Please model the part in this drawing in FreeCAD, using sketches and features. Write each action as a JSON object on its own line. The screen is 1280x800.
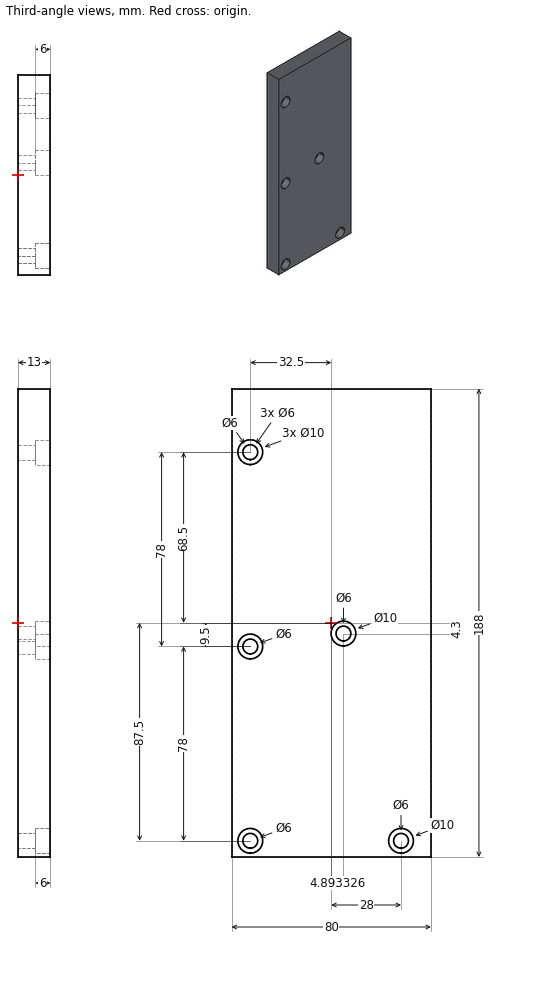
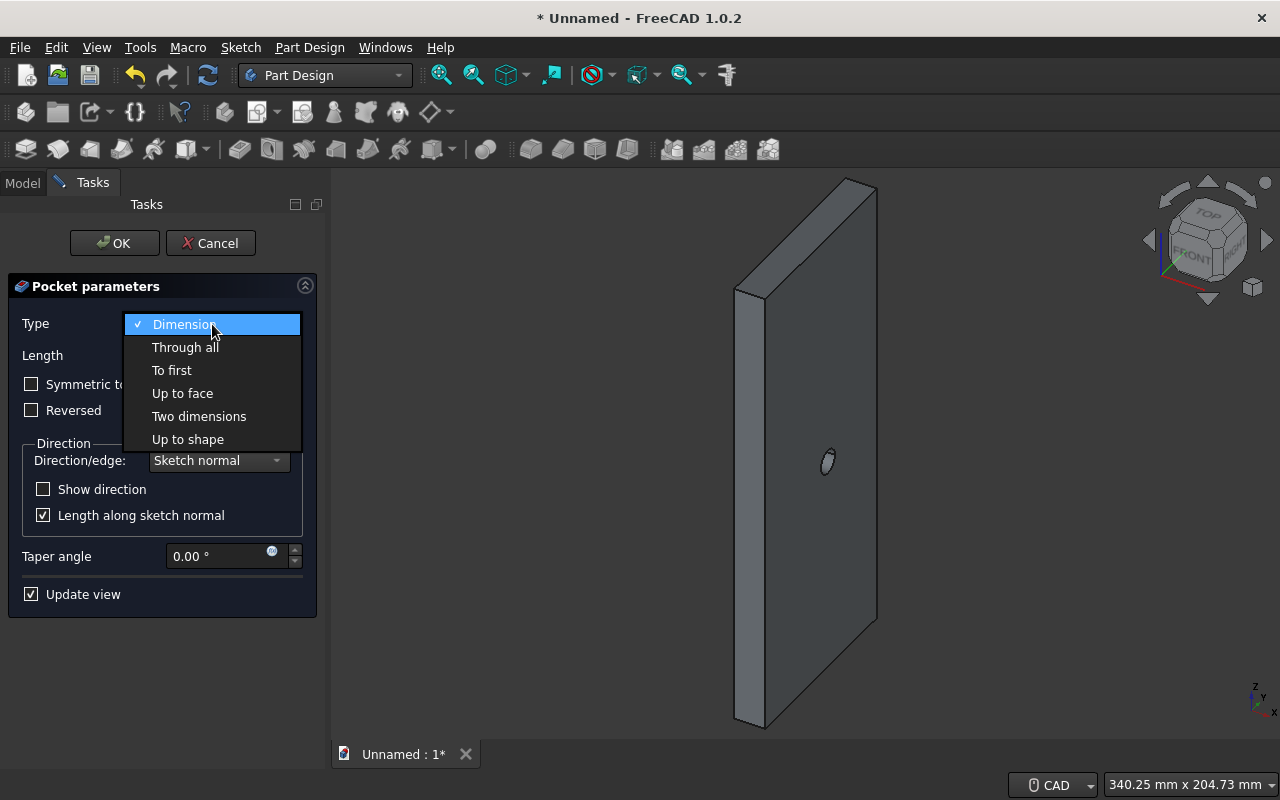
{"action": "left_click", "coordinate": [212, 370]}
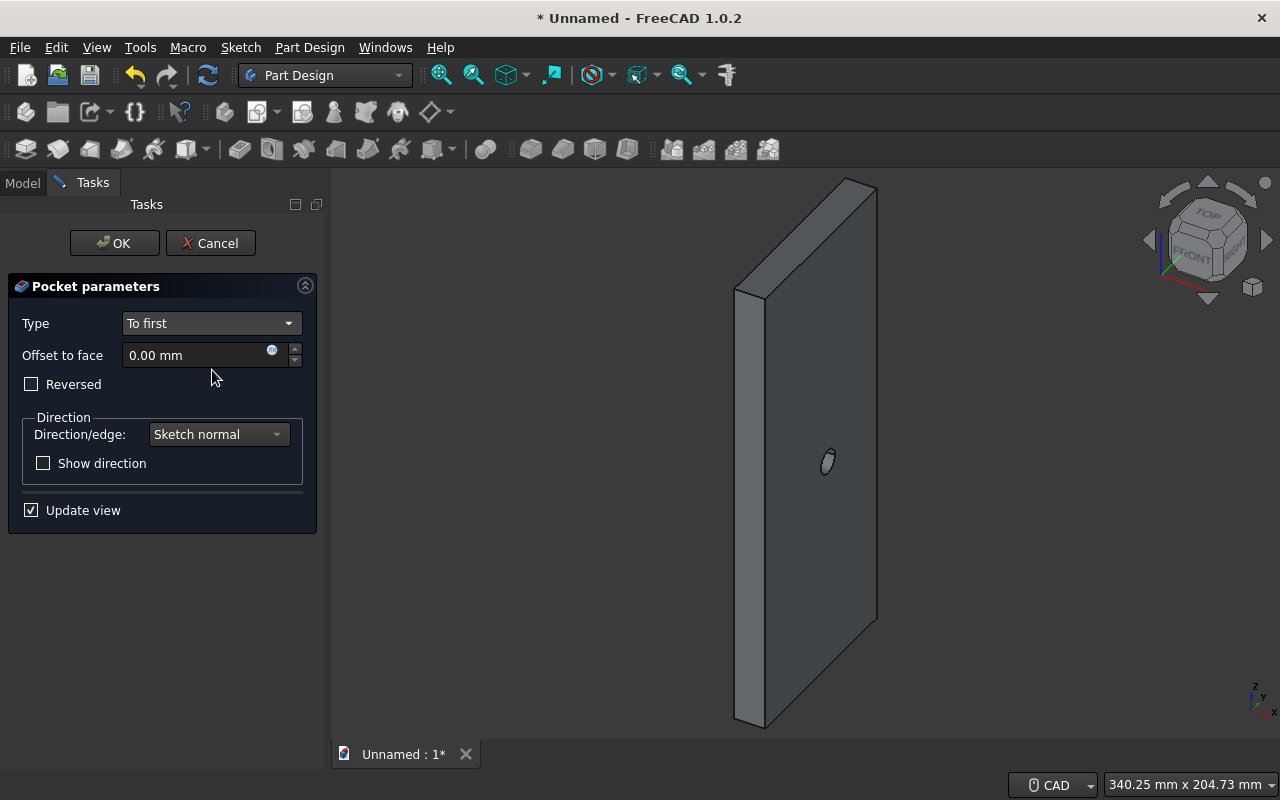
{"action": "left_click", "coordinate": [115, 243]}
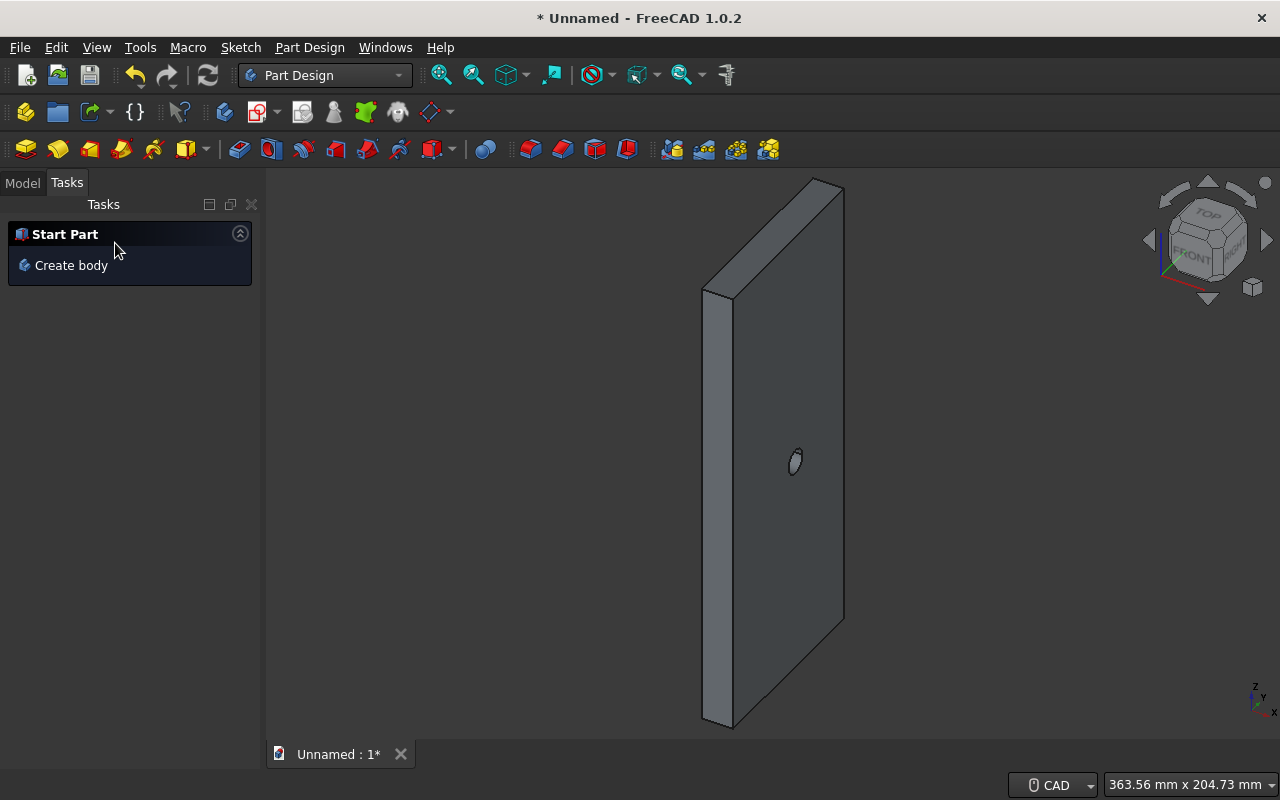
{"action": "left_click", "coordinate": [789, 580]}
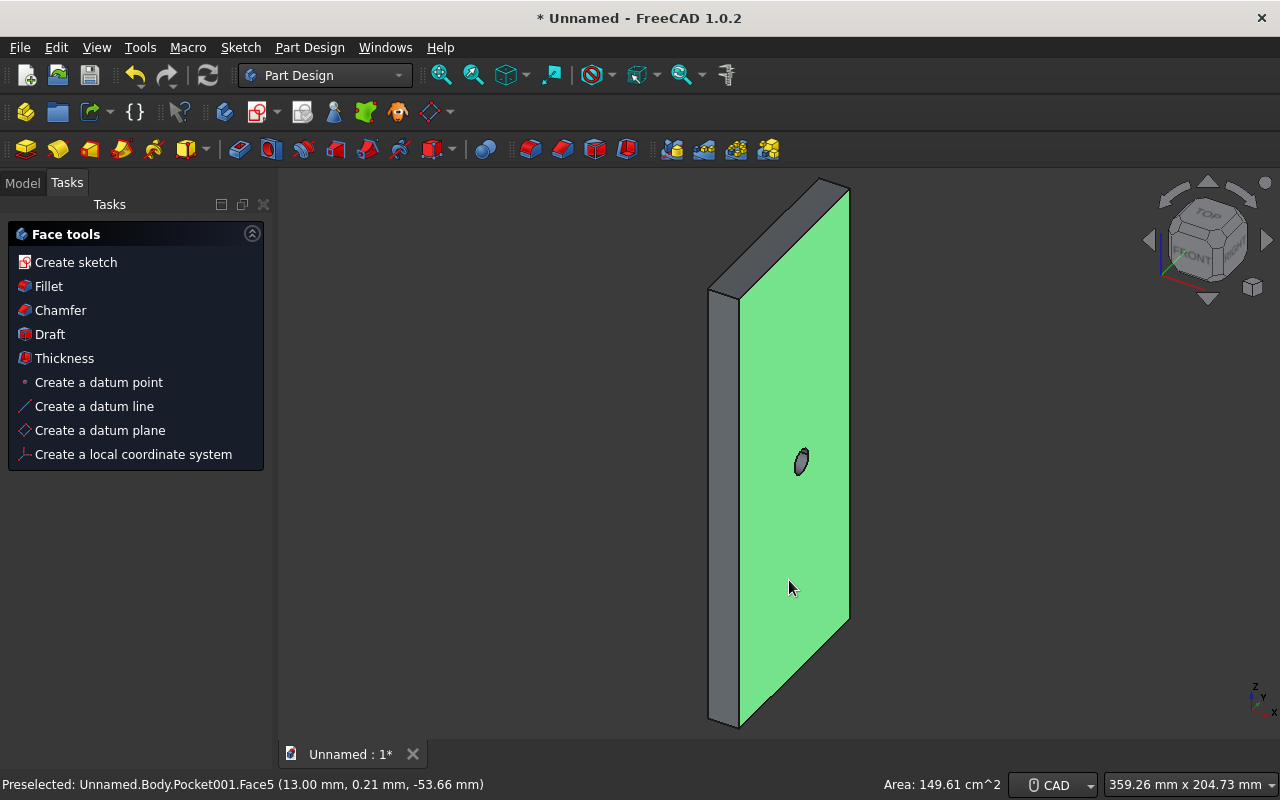
{"action": "left_click", "coordinate": [258, 112]}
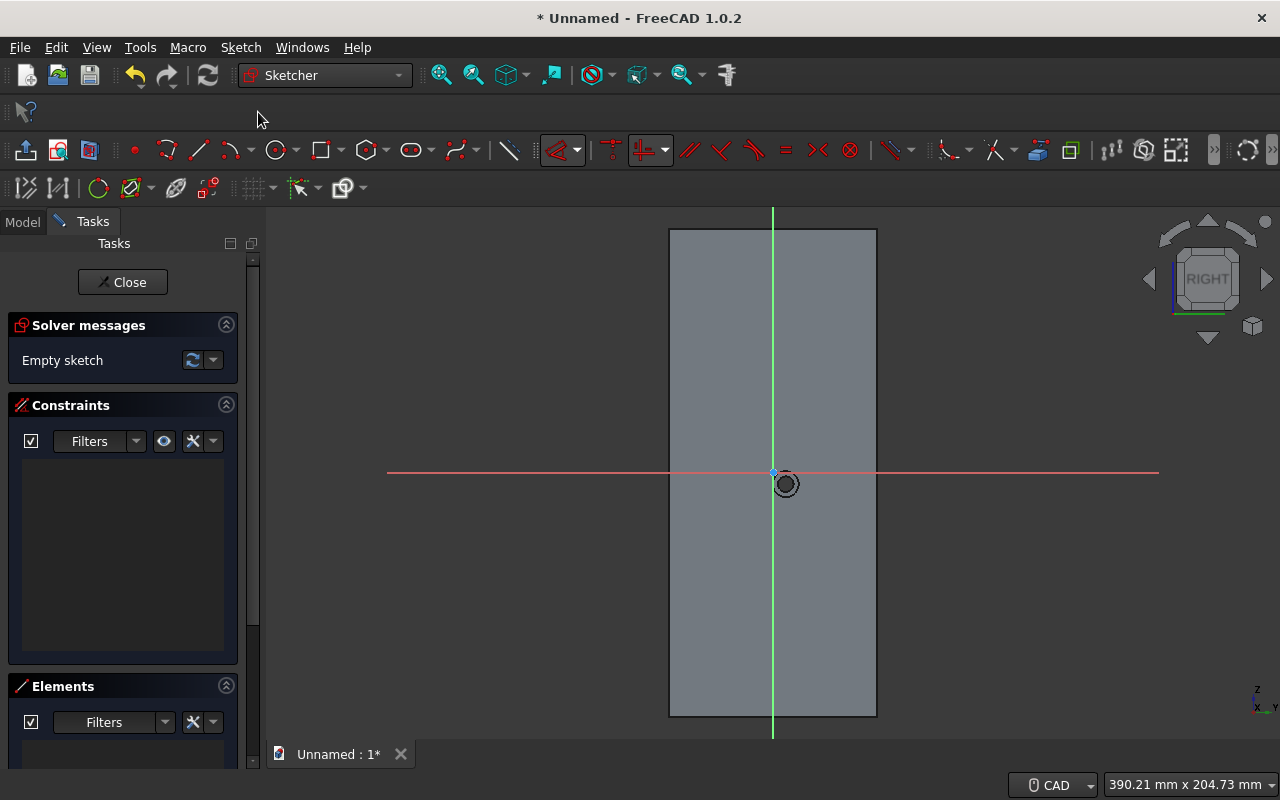
{"action": "scroll", "coordinate": [615, 361], "scroll_direction": "down", "scroll_amount": 1}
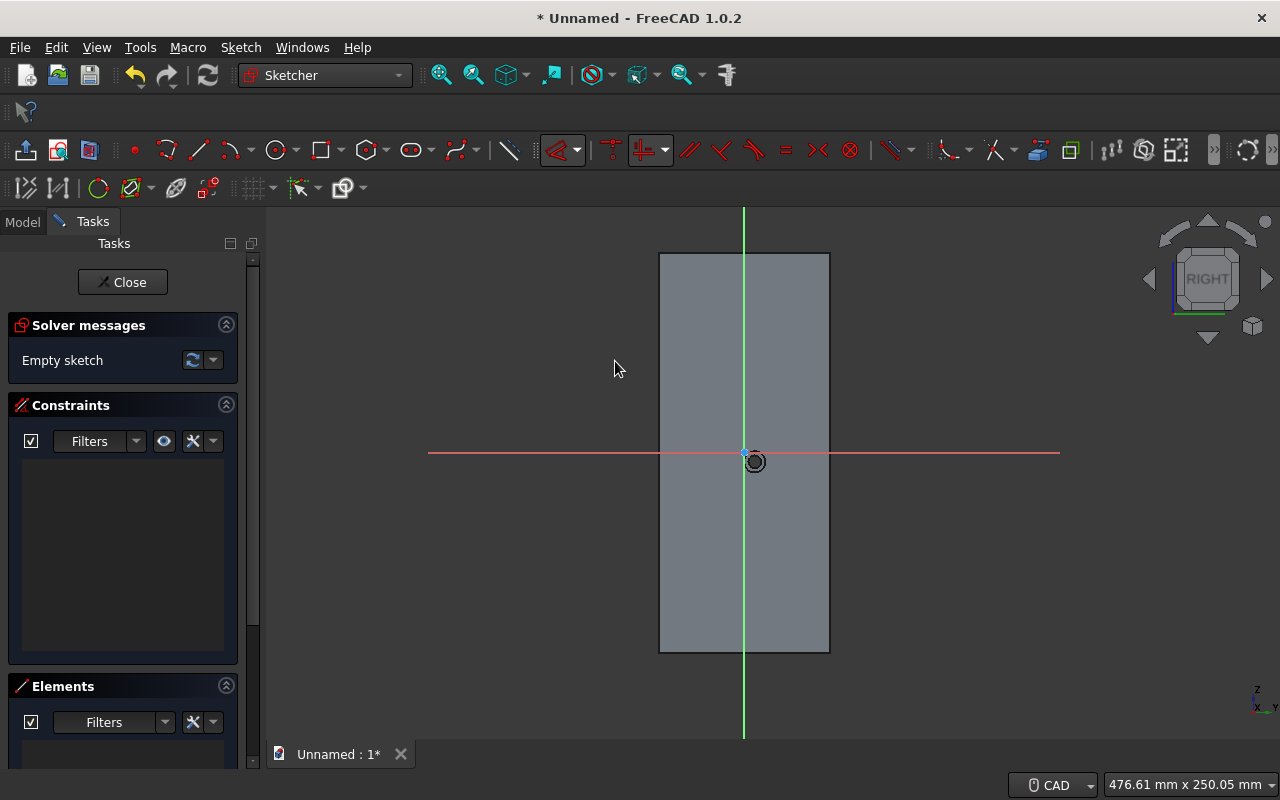
{"action": "key", "text": "g c"}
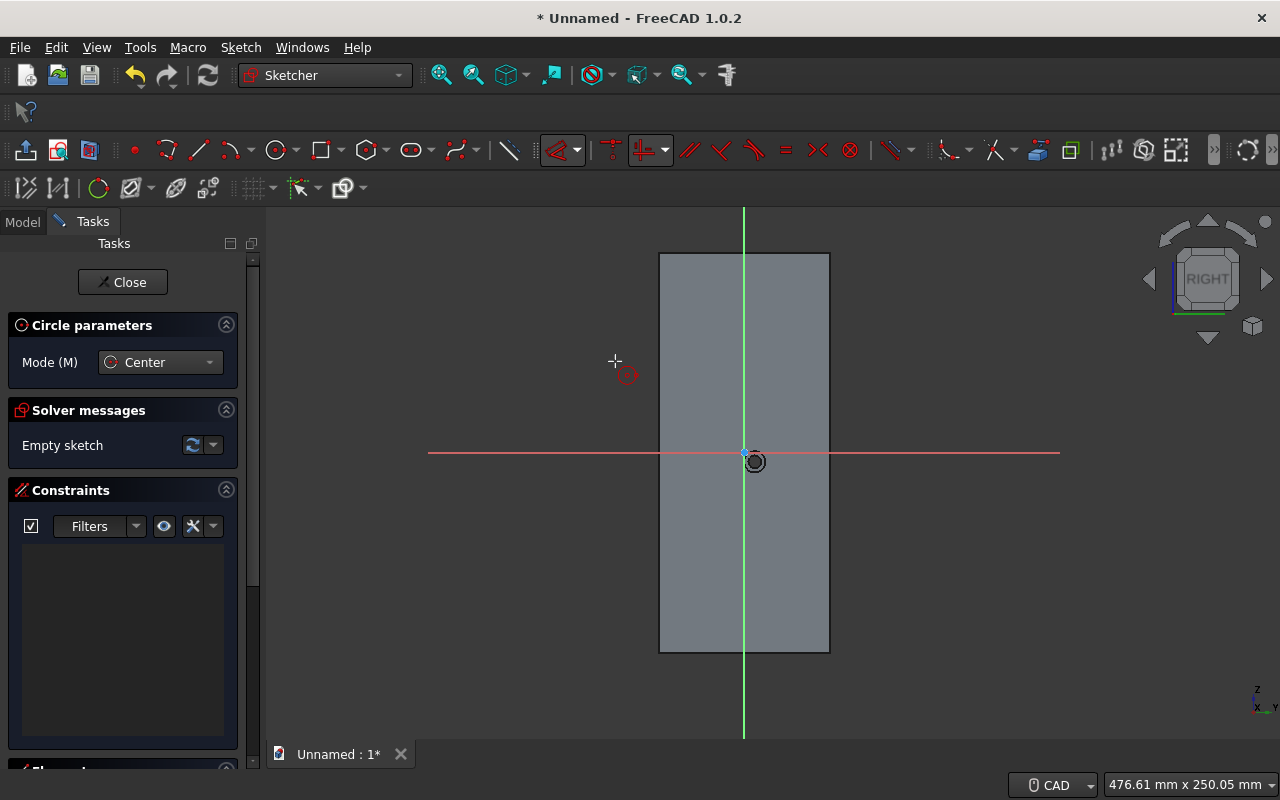
{"action": "scroll", "coordinate": [675, 307], "scroll_direction": "up", "scroll_amount": 4}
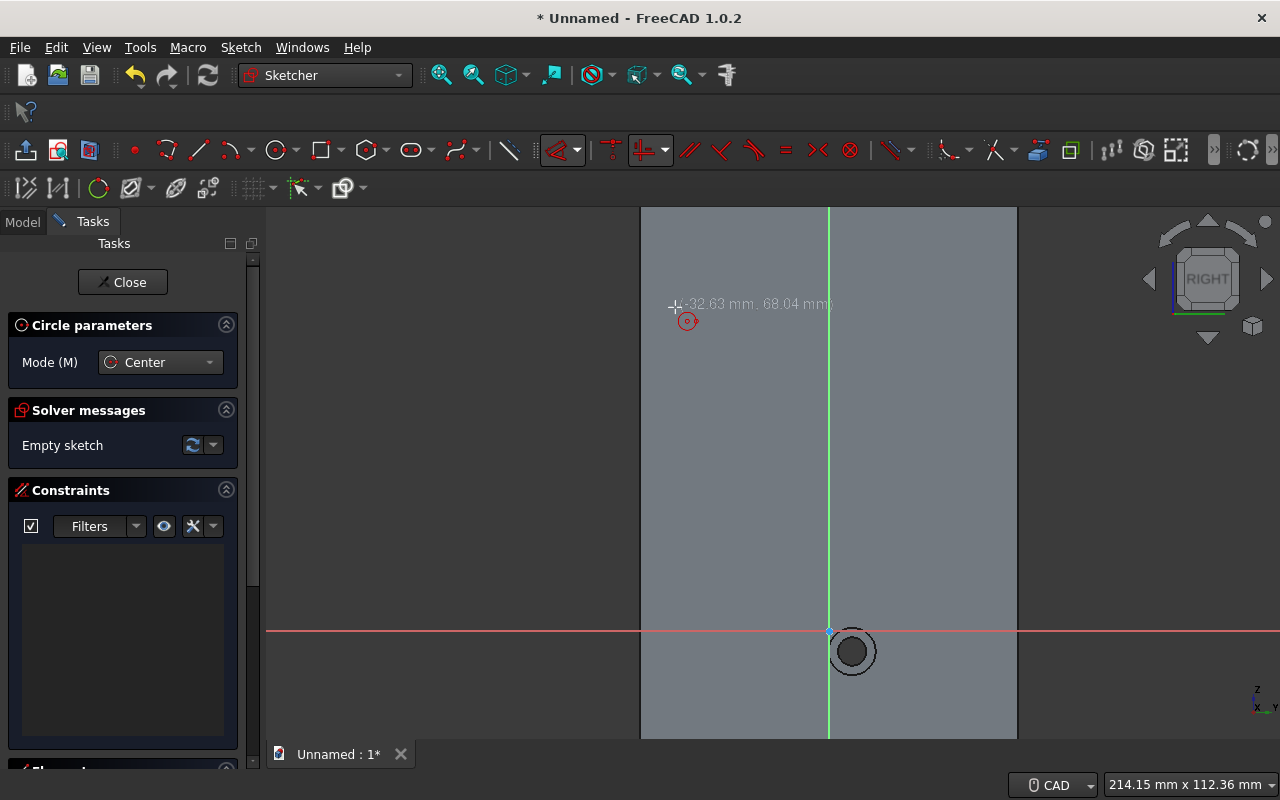
{"action": "left_click", "coordinate": [675, 307]}
{"action": "left_click", "coordinate": [692, 290]}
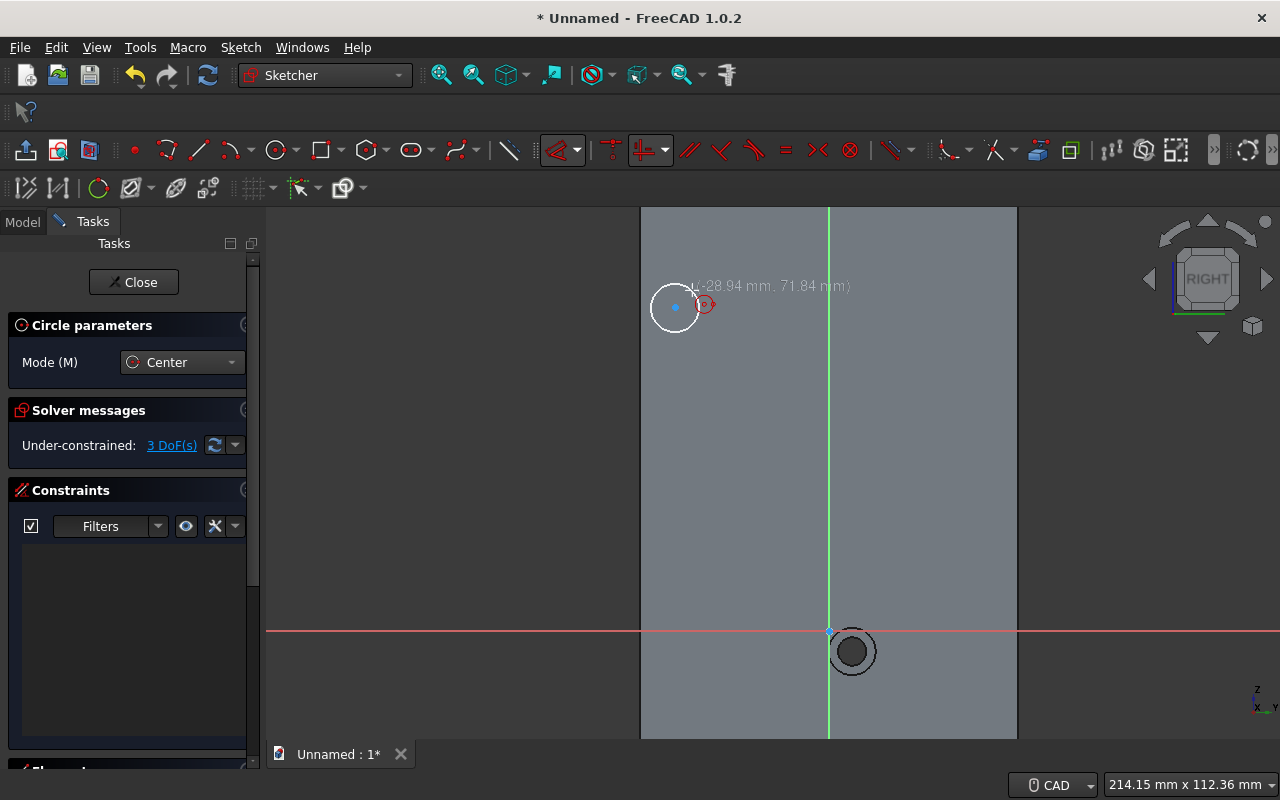
{"action": "left_click", "coordinate": [675, 676]}
{"action": "left_click", "coordinate": [692, 659]}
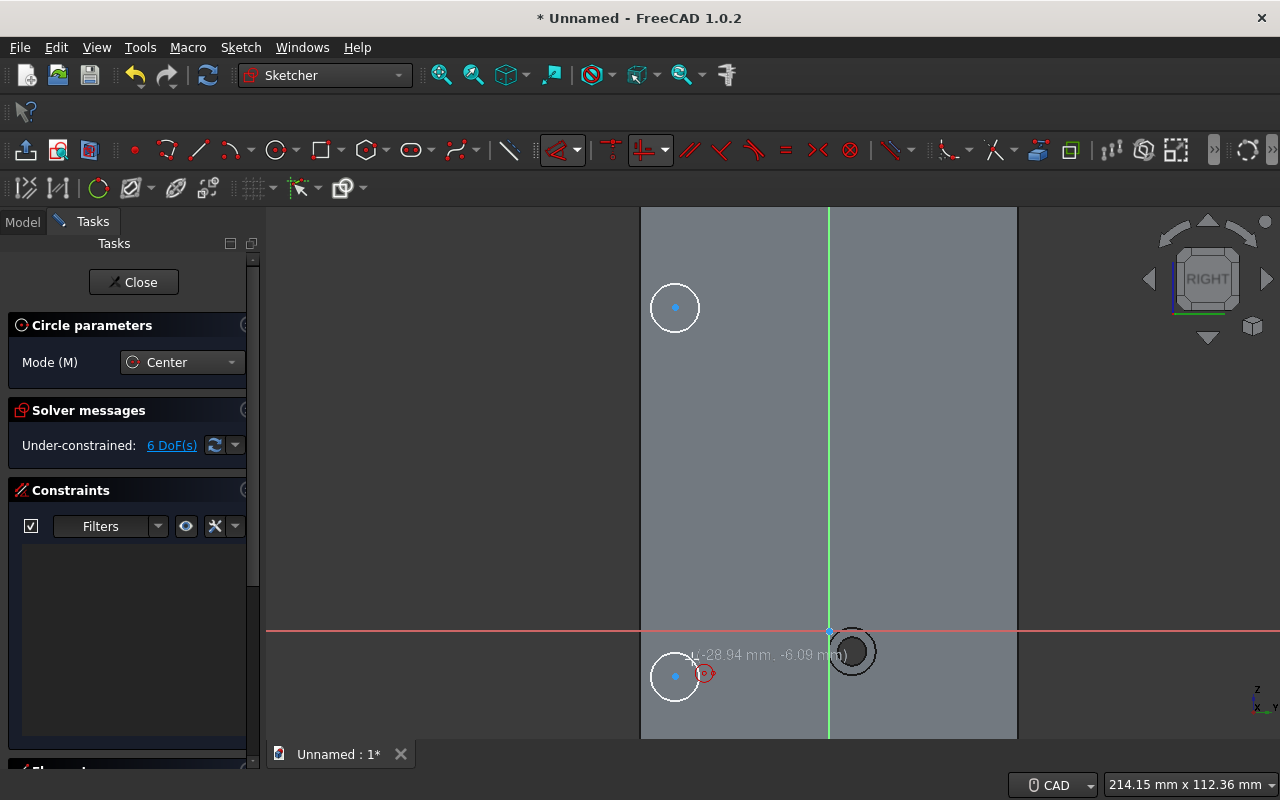
{"action": "scroll", "coordinate": [675, 307], "scroll_direction": "down", "scroll_amount": 4}